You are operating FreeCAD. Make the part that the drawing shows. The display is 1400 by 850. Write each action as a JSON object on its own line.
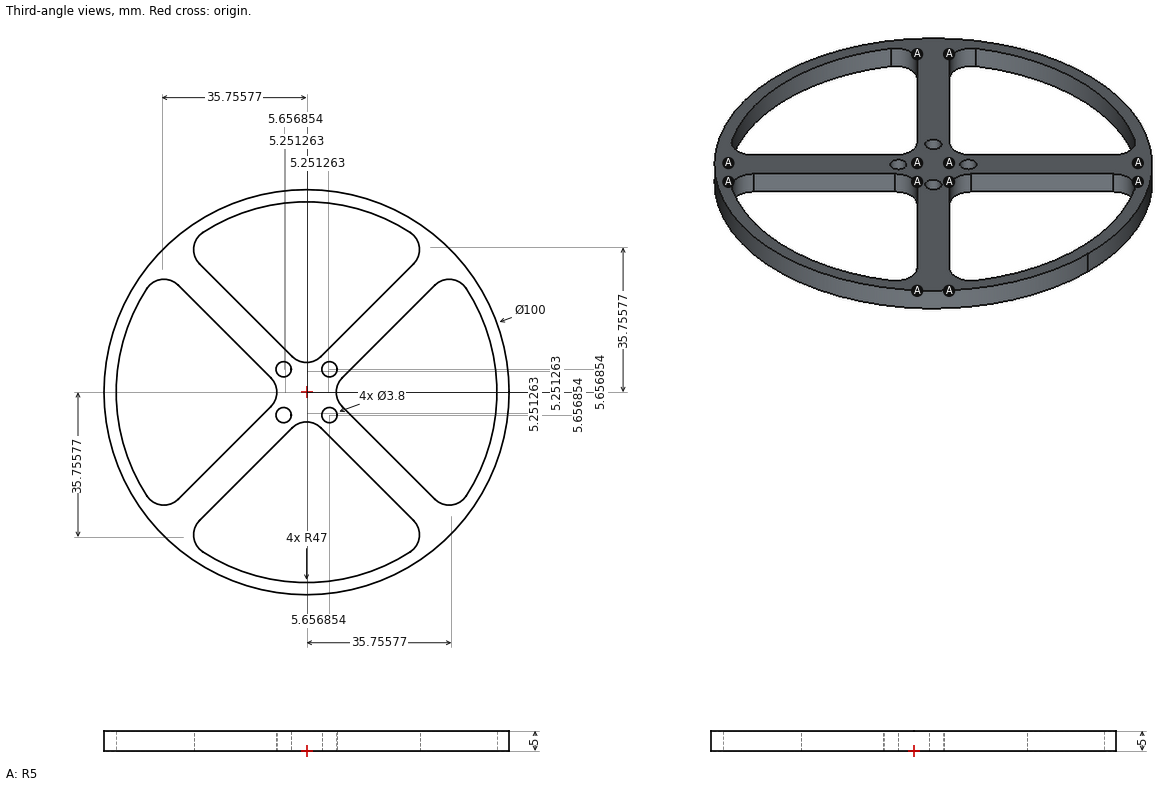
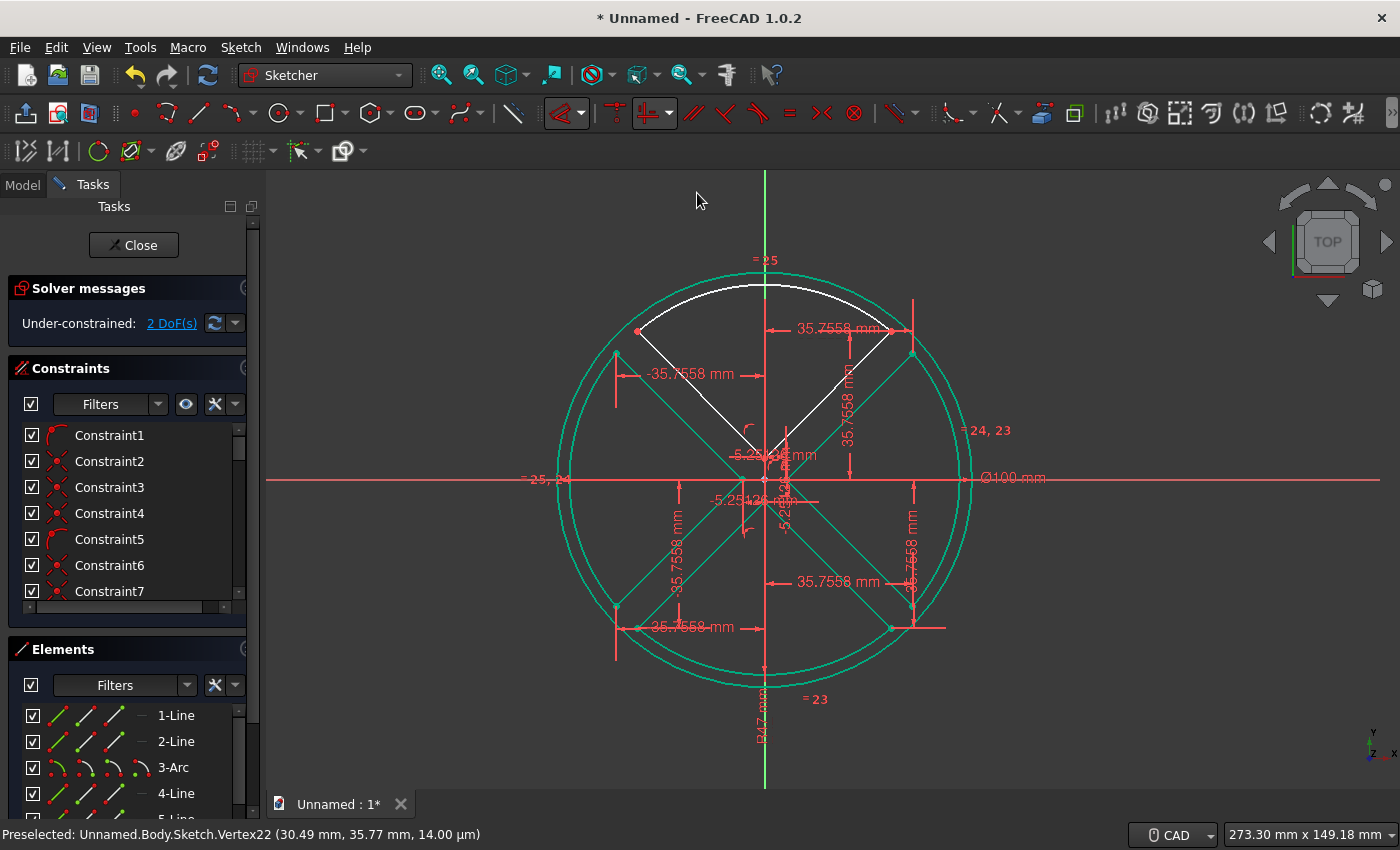
{"action": "scroll", "coordinate": [765, 459], "scroll_direction": "up", "scroll_amount": 3}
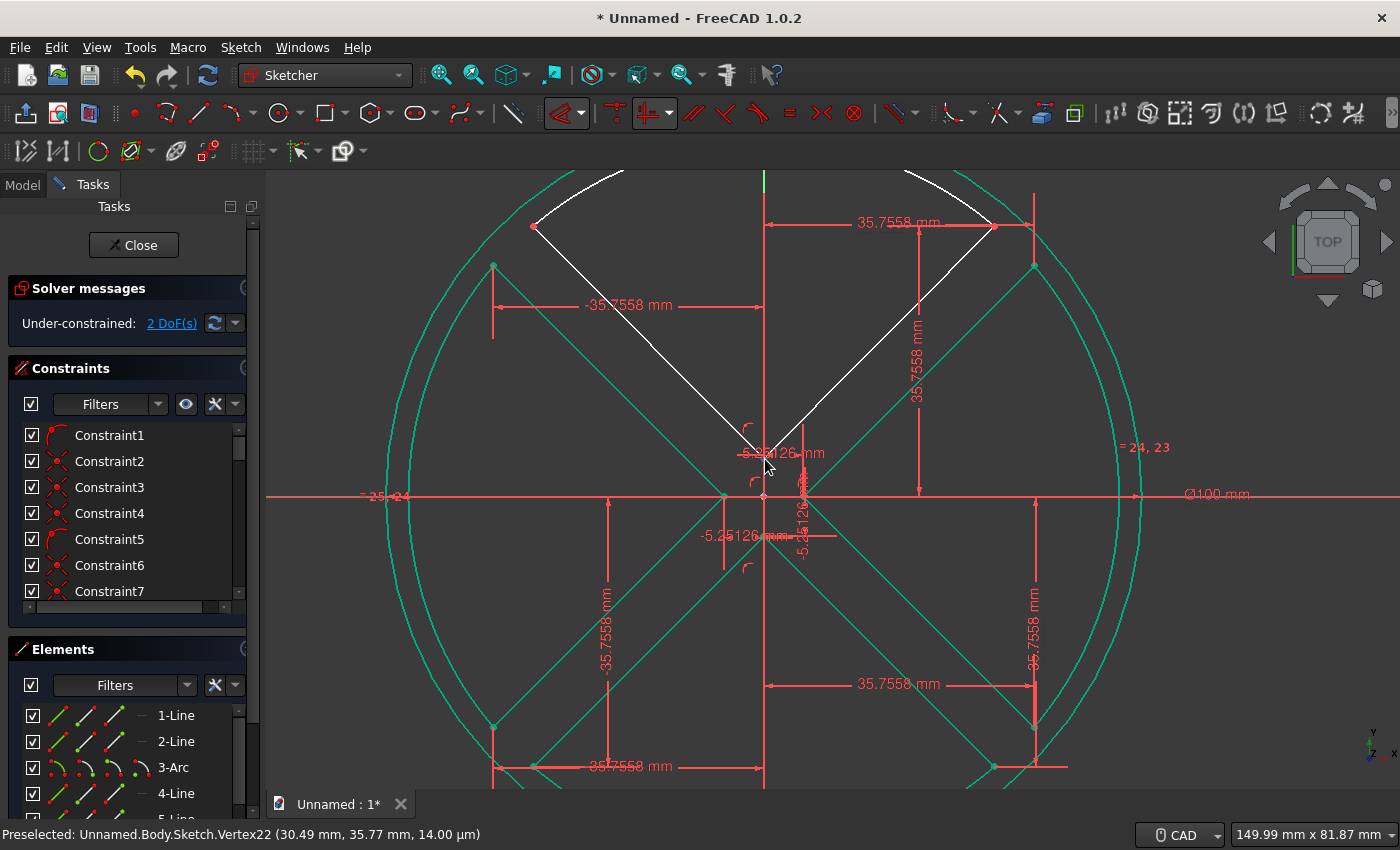
{"action": "left_click", "coordinate": [764, 459]}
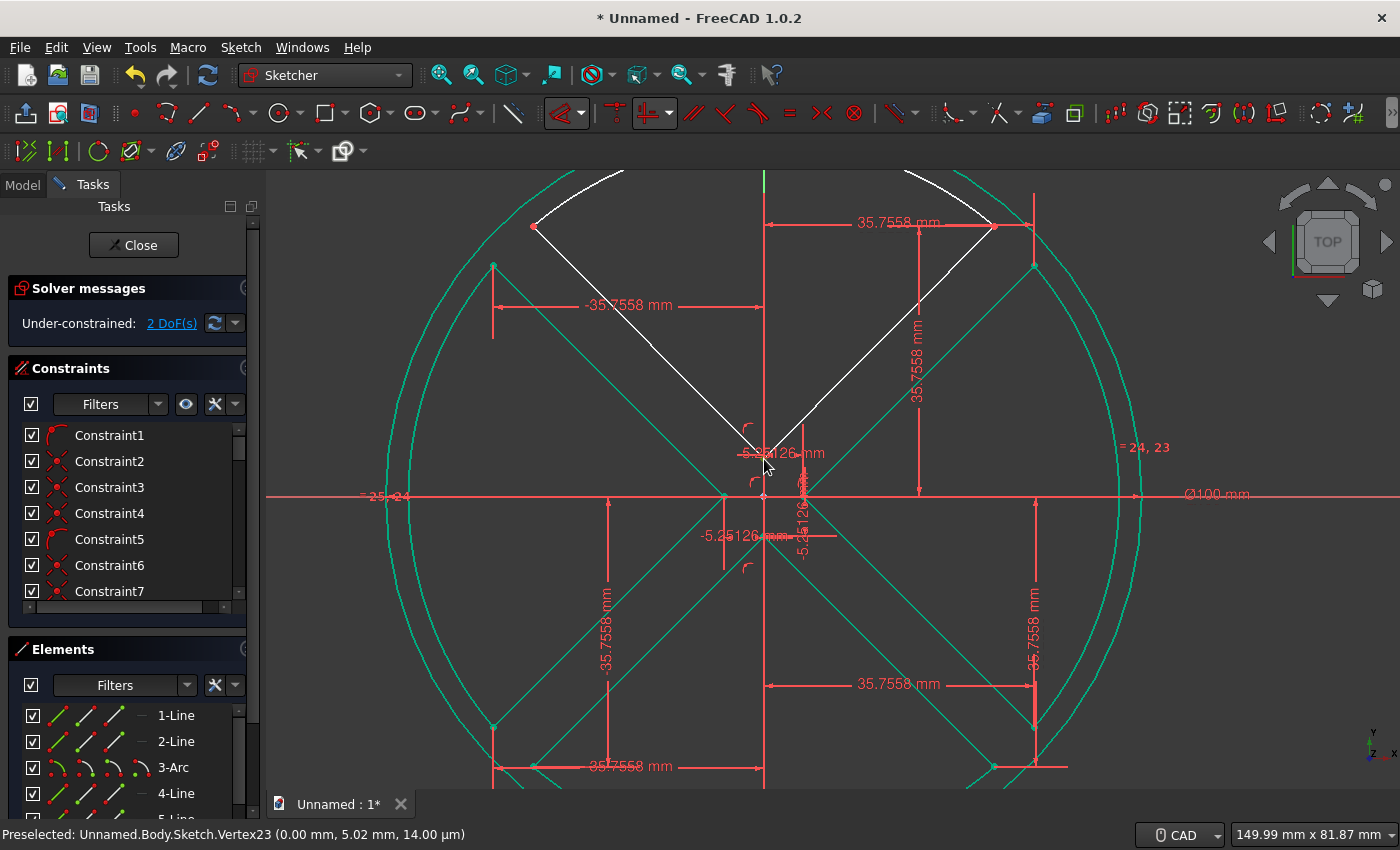
{"action": "key", "text": "i"}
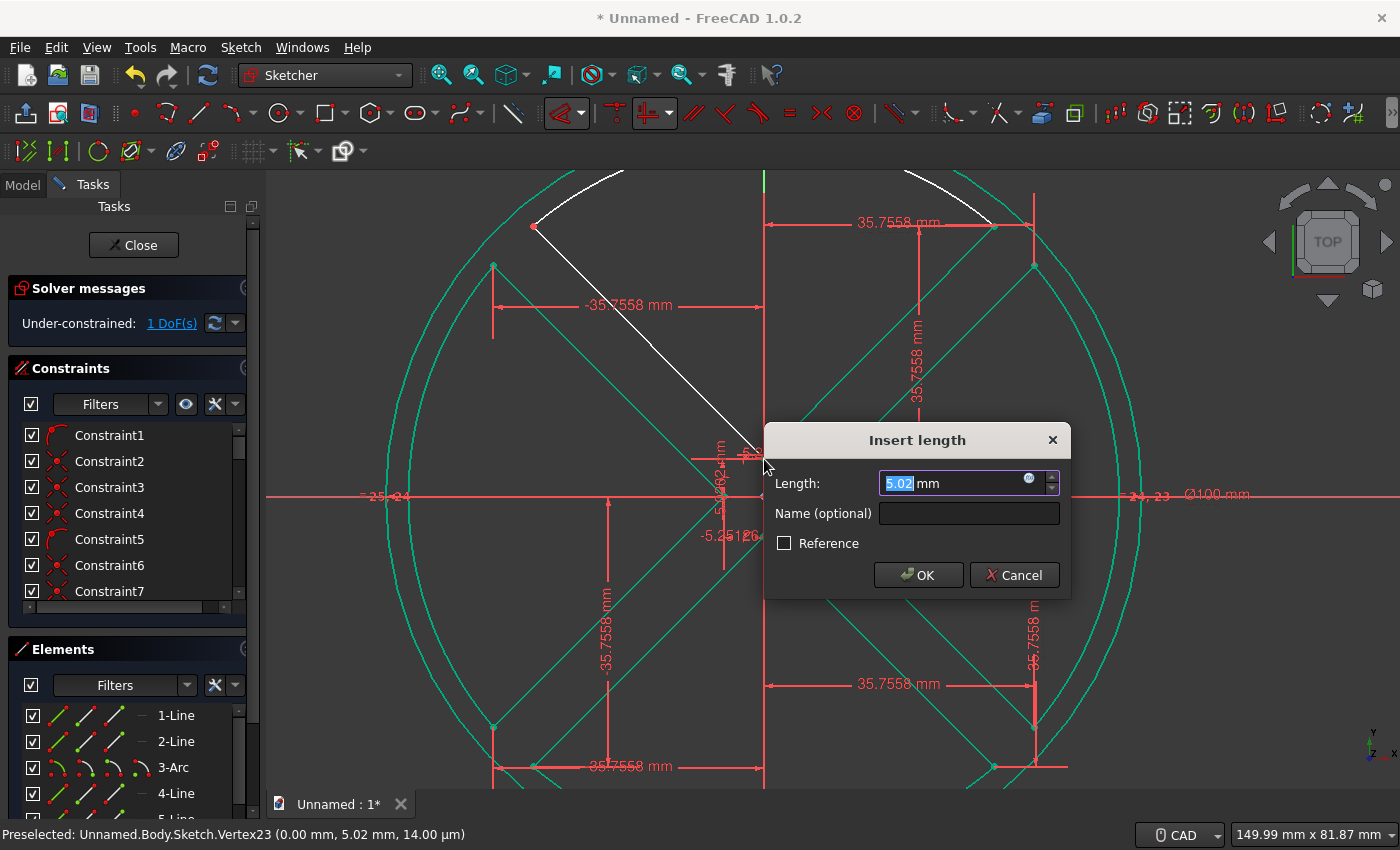
{"action": "type", "text": "5.251263"}
{"action": "key", "text": "Return"}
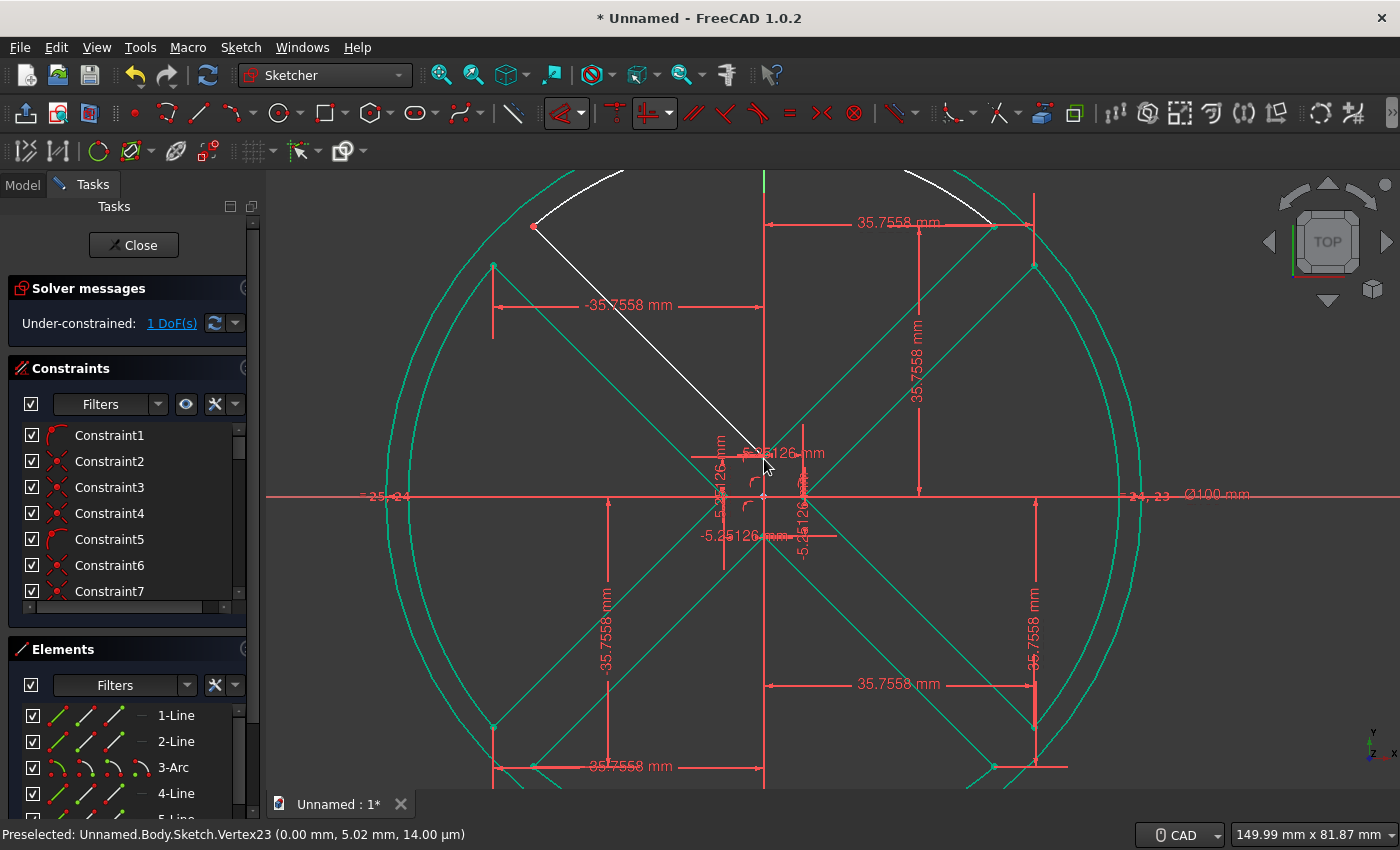
{"action": "left_click", "coordinate": [533, 226]}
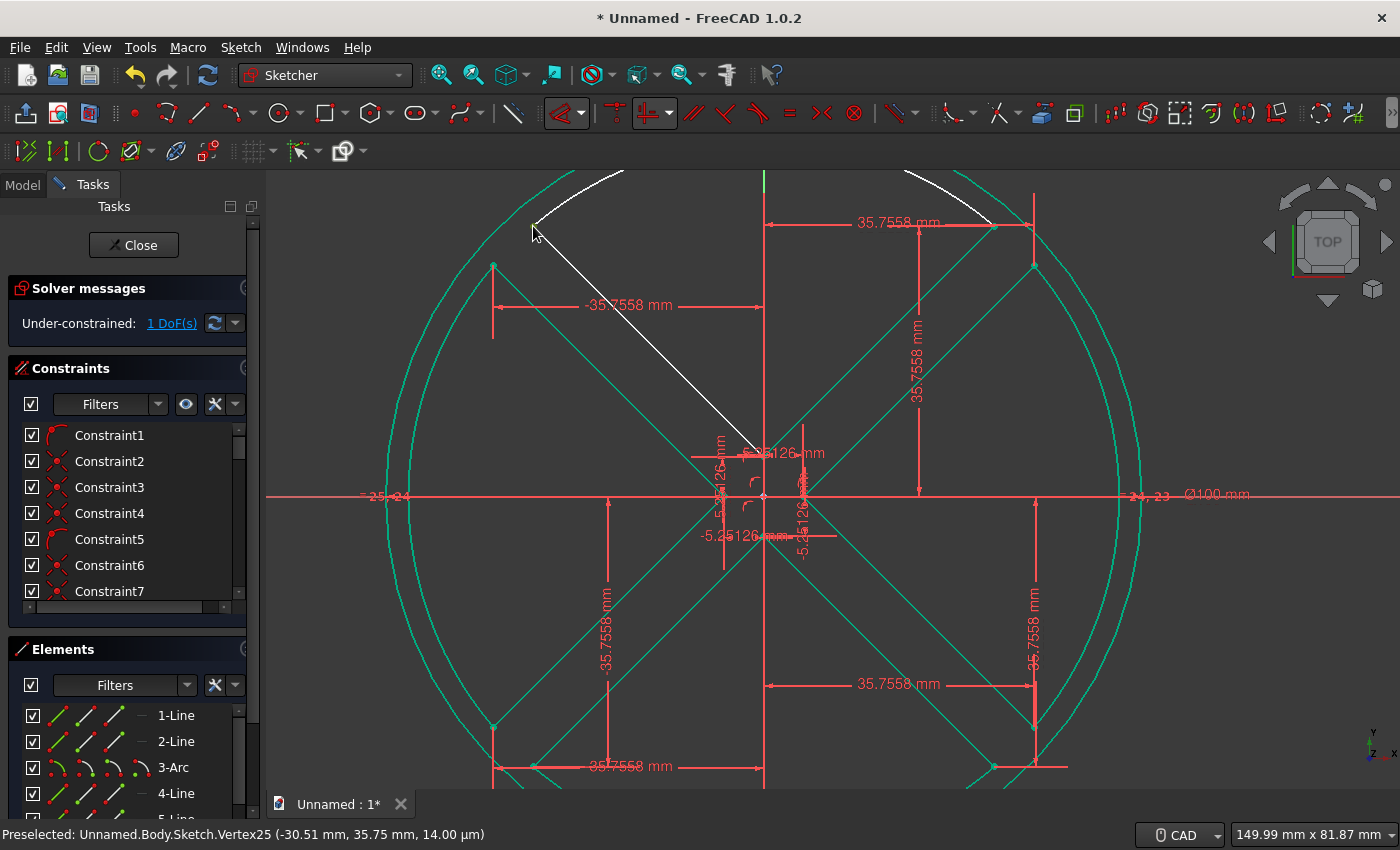
{"action": "left_click", "coordinate": [584, 114]}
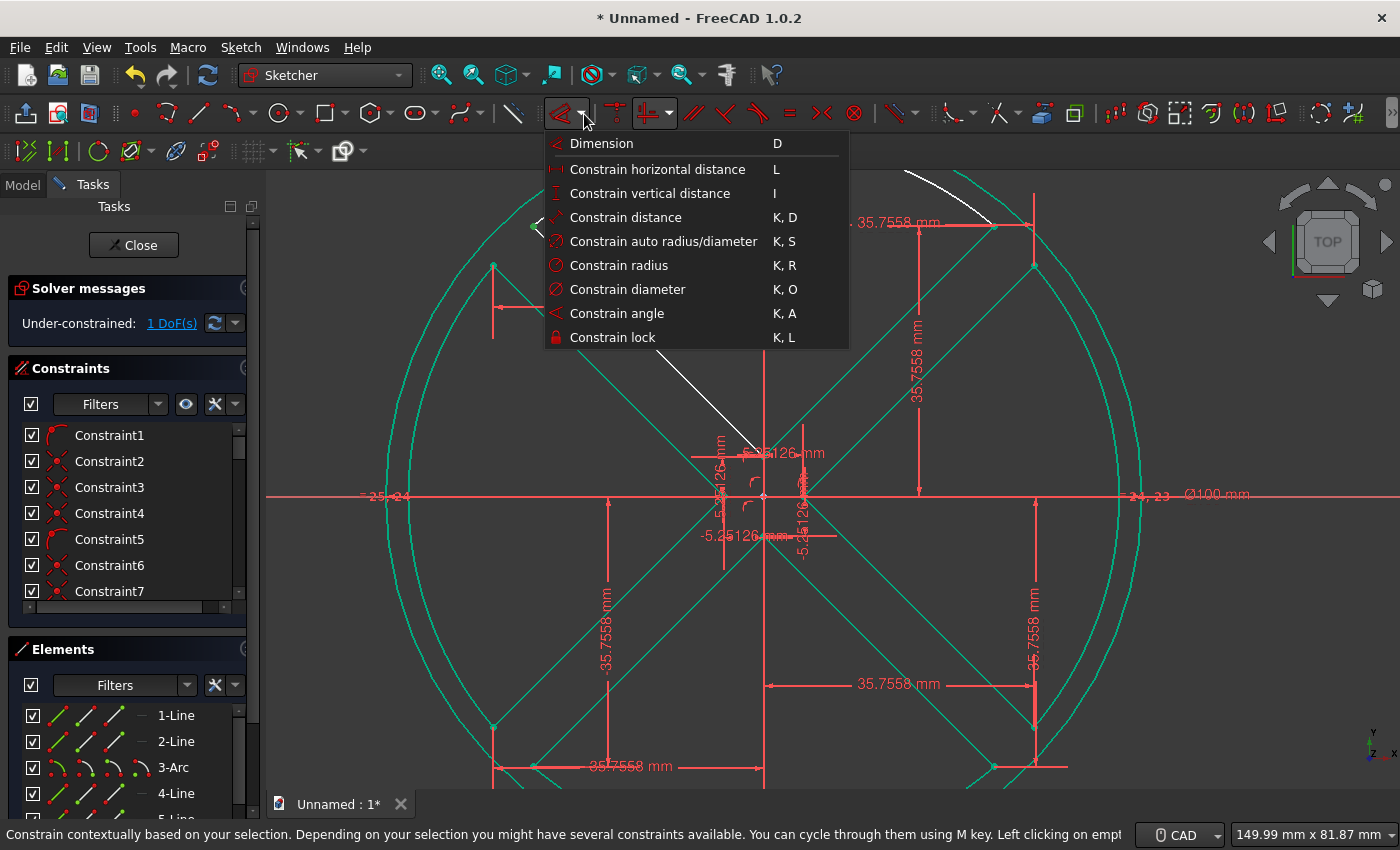
{"action": "left_click", "coordinate": [697, 193]}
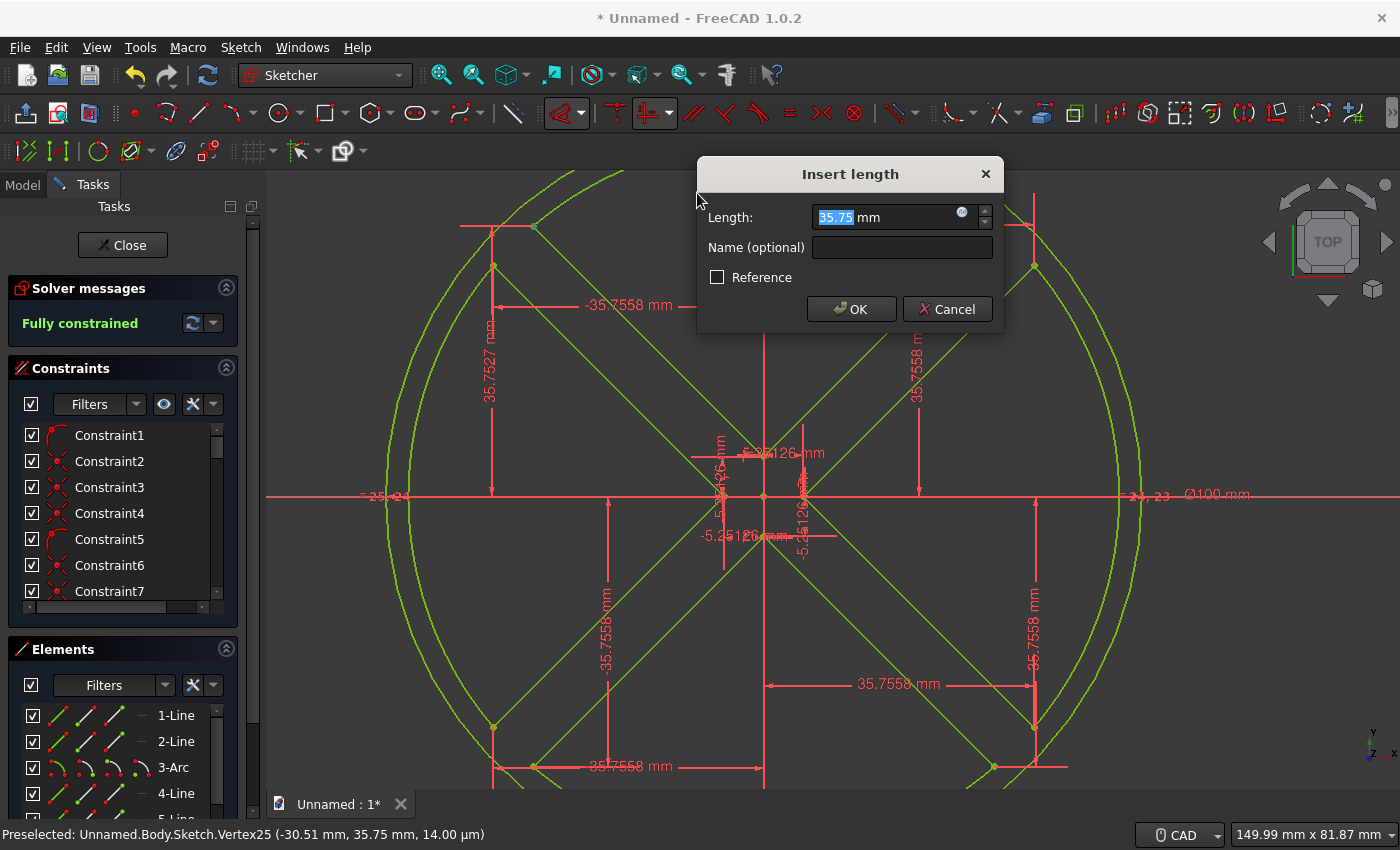
{"action": "type", "text": "35.75577"}
{"action": "key", "text": "Return"}